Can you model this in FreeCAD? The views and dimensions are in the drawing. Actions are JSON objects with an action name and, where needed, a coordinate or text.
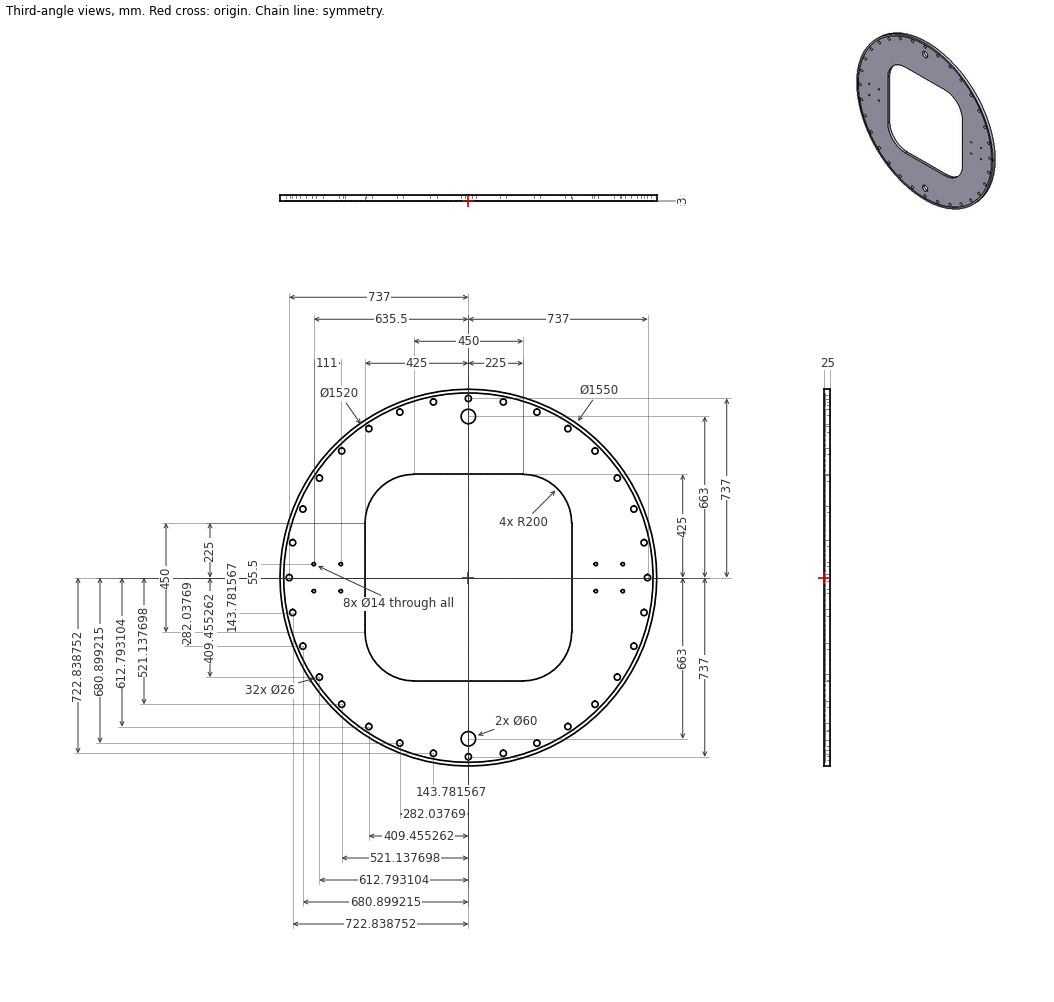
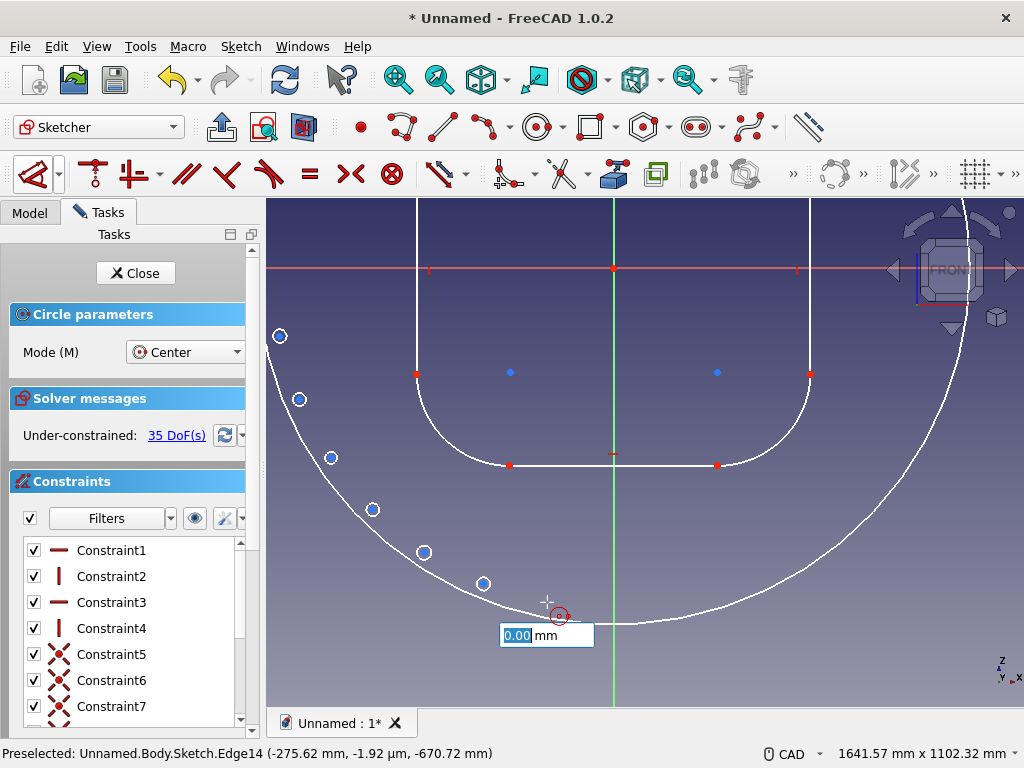
{"action": "scroll", "coordinate": [551, 598], "scroll_direction": "up", "scroll_amount": 5}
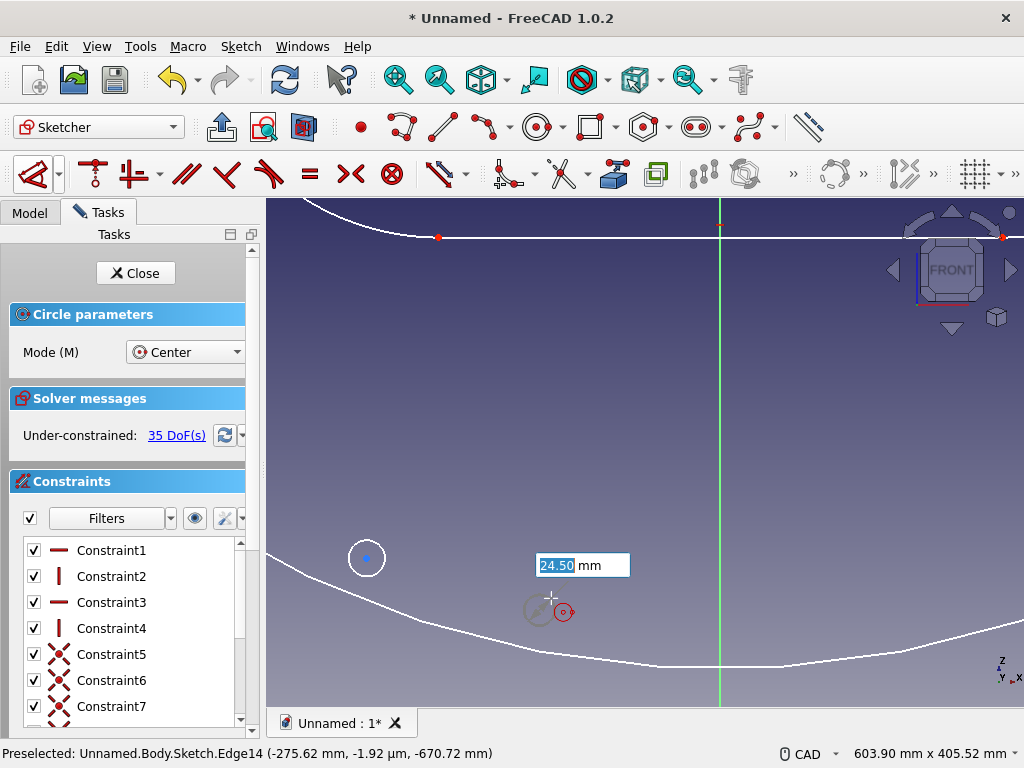
{"action": "left_click", "coordinate": [552, 596]}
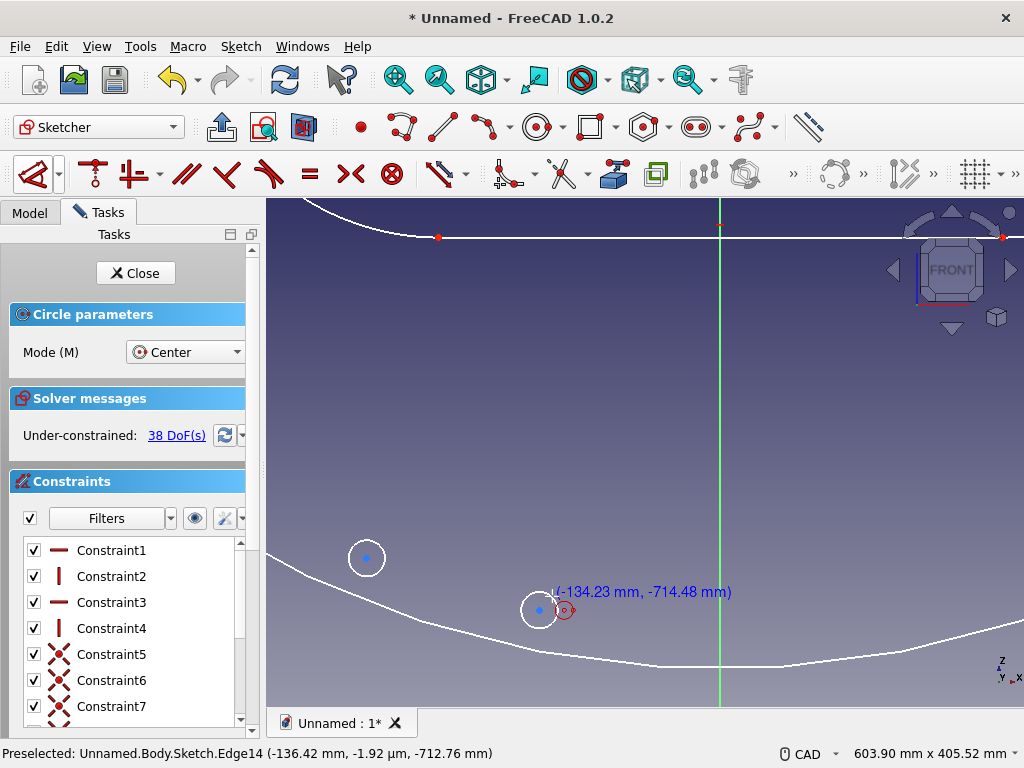
{"action": "scroll", "coordinate": [720, 625], "scroll_direction": "up", "scroll_amount": 2}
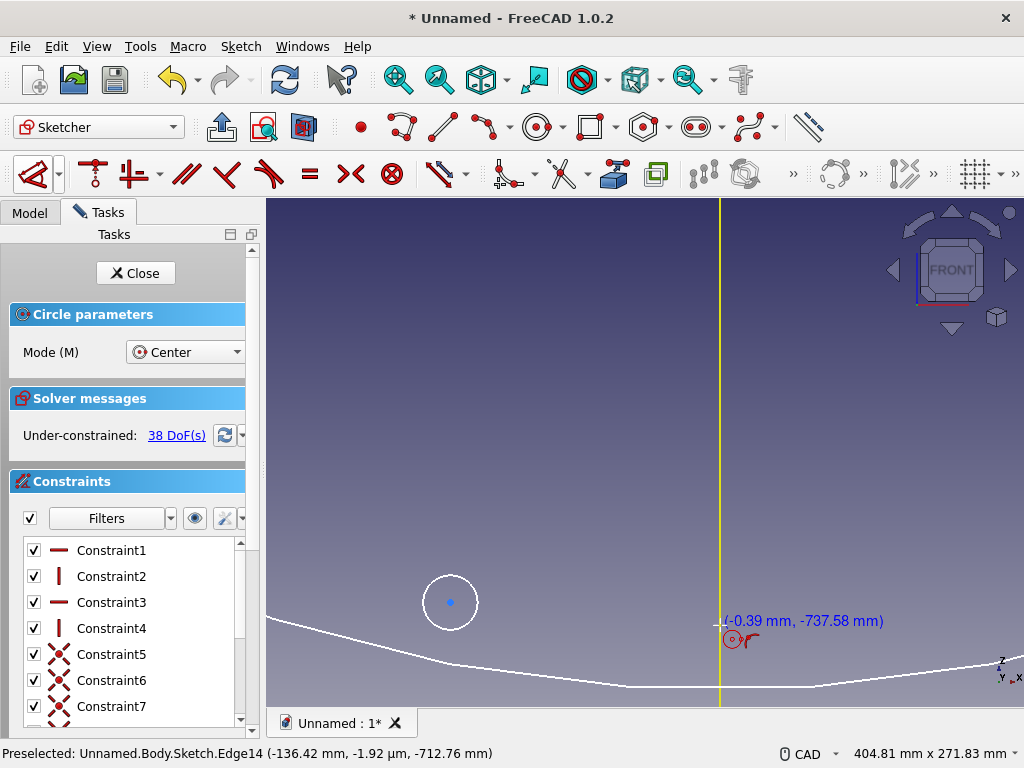
{"action": "scroll", "coordinate": [559, 603], "scroll_direction": "down", "scroll_amount": 11}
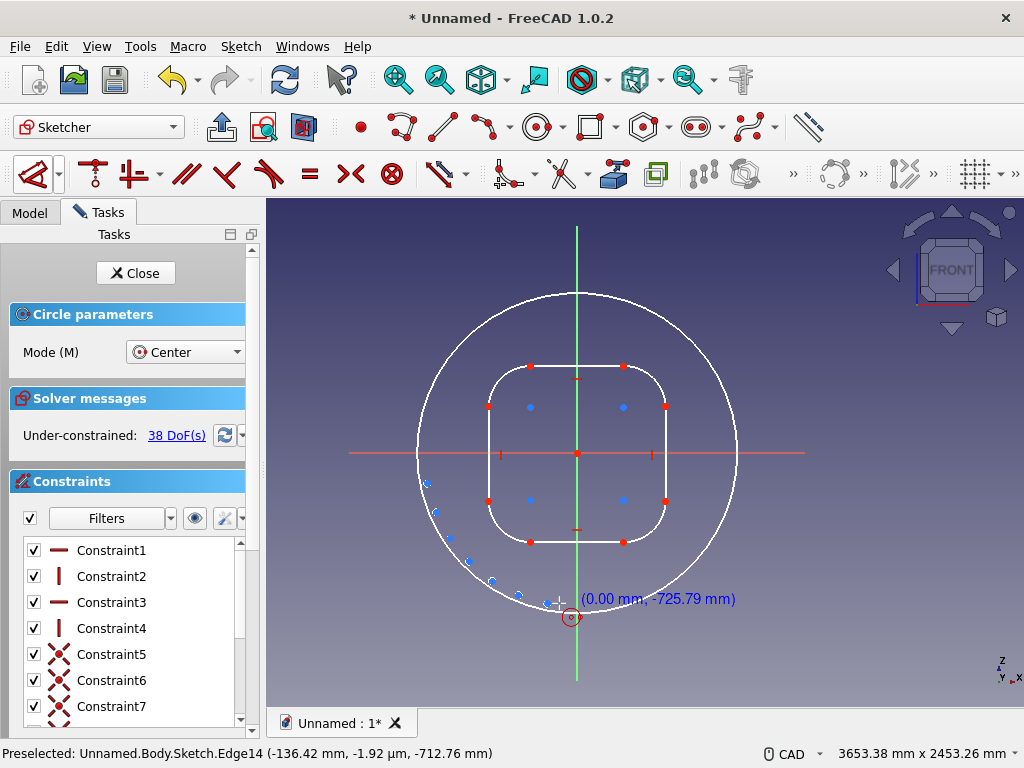
{"action": "scroll", "coordinate": [577, 606], "scroll_direction": "up", "scroll_amount": 4}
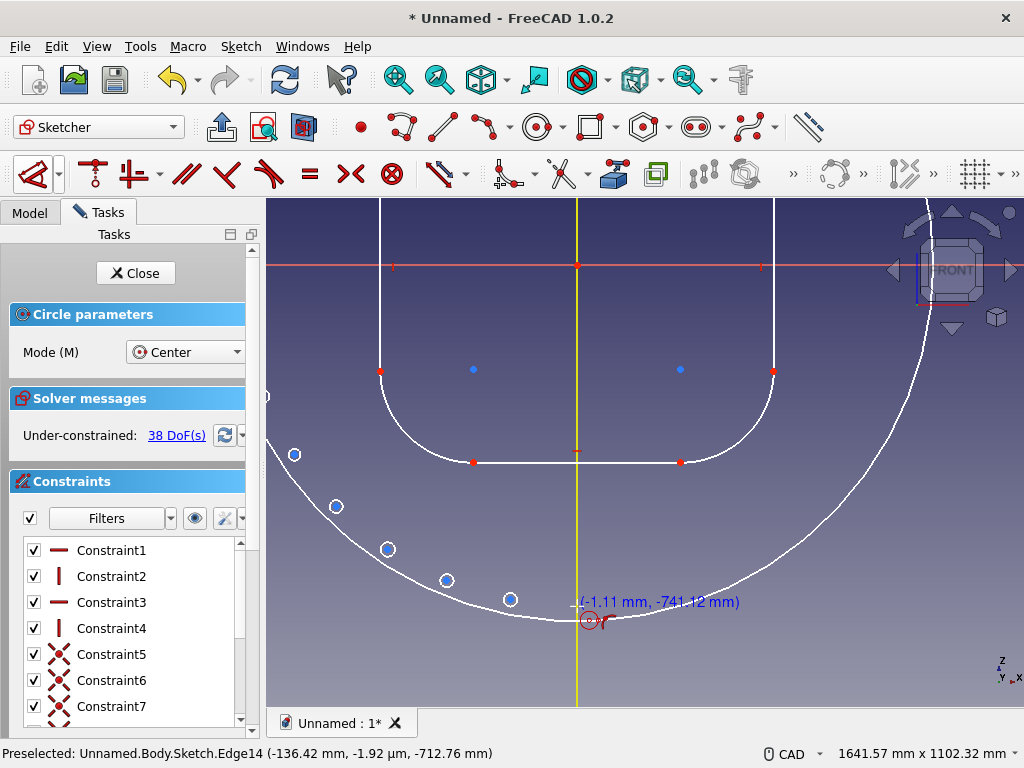
{"action": "left_click", "coordinate": [577, 605]}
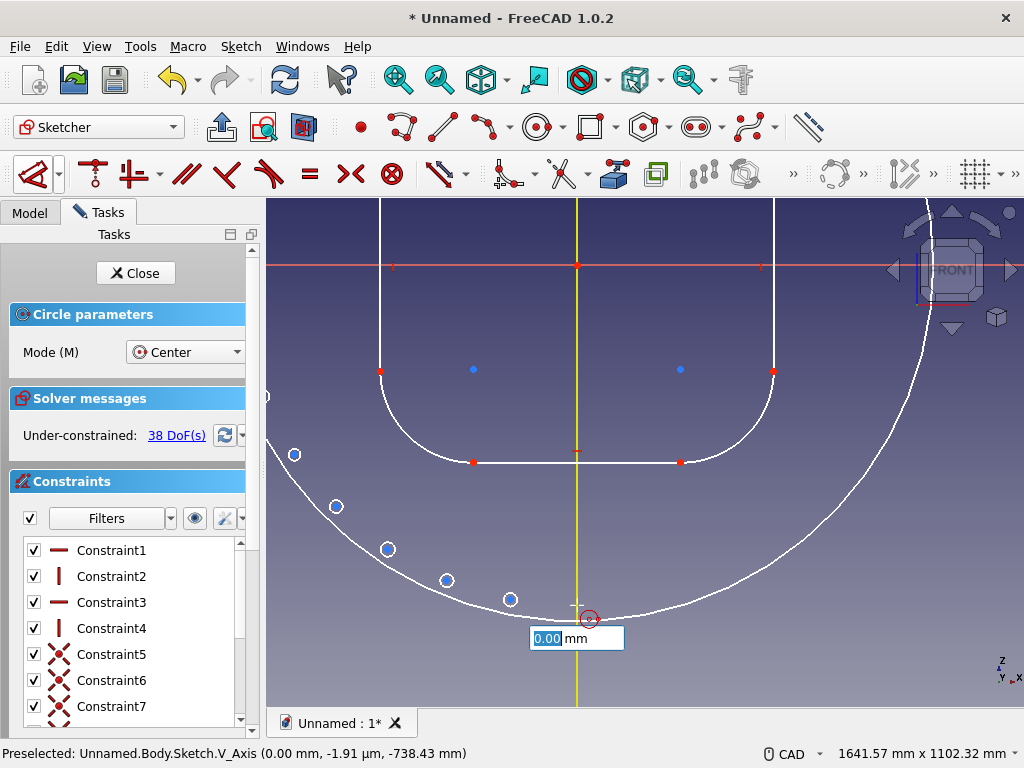
{"action": "scroll", "coordinate": [583, 603], "scroll_direction": "up", "scroll_amount": 6}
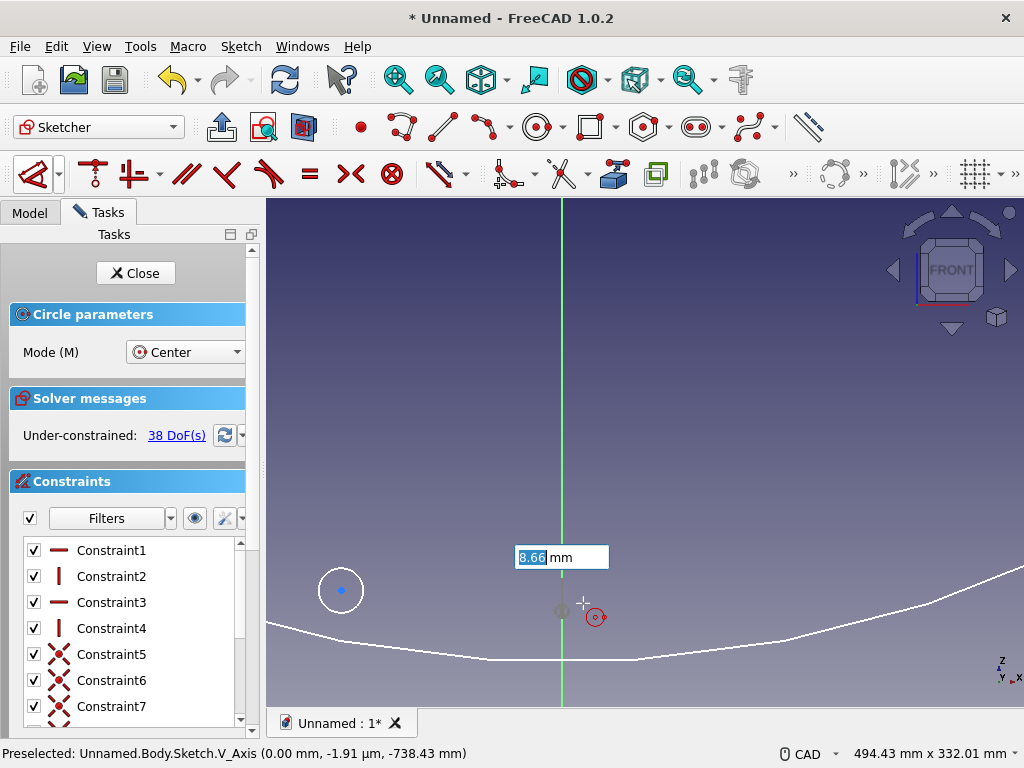
{"action": "left_click", "coordinate": [581, 602]}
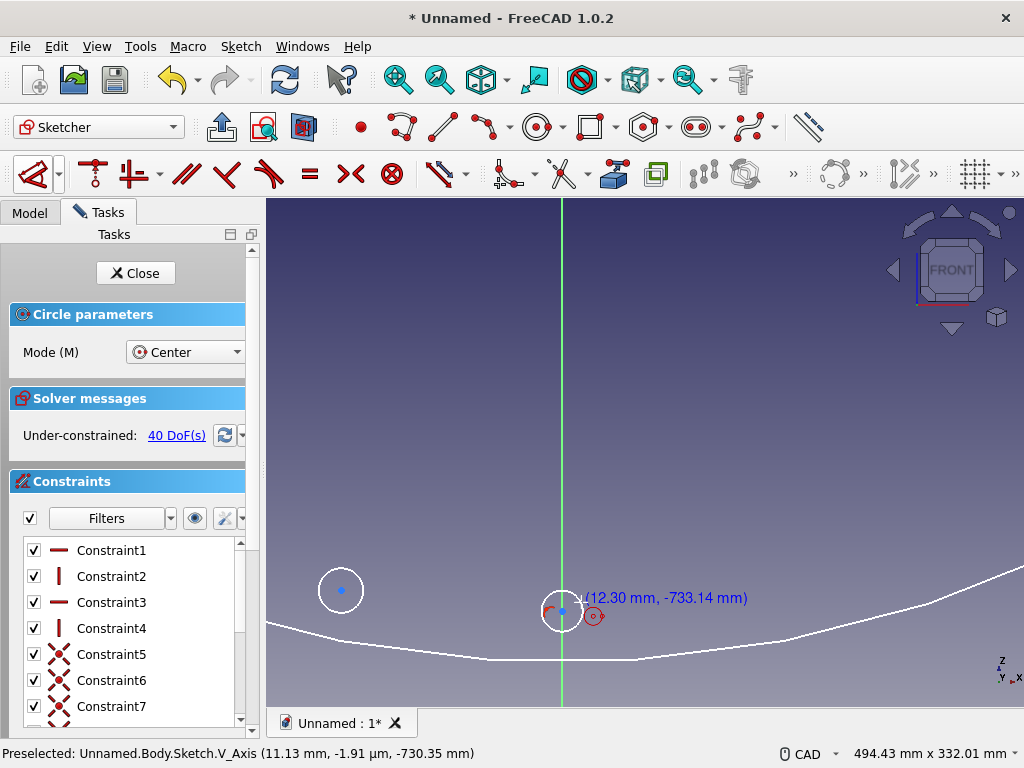
{"action": "scroll", "coordinate": [579, 605], "scroll_direction": "down", "scroll_amount": 10}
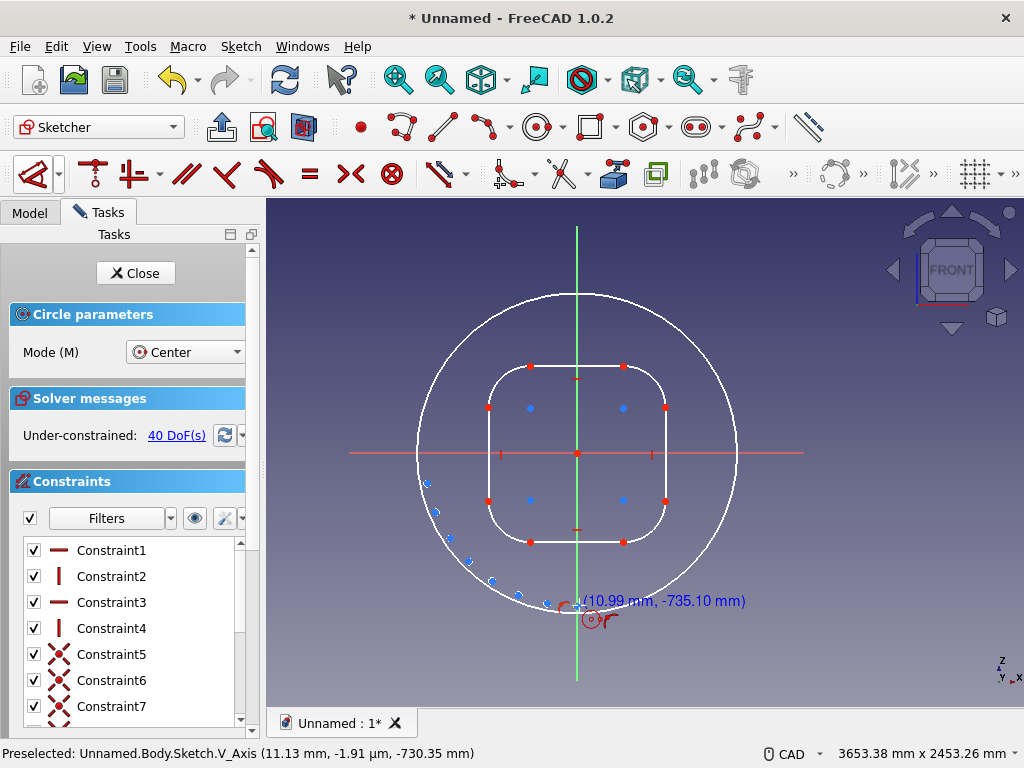
{"action": "scroll", "coordinate": [577, 591], "scroll_direction": "up", "scroll_amount": 2}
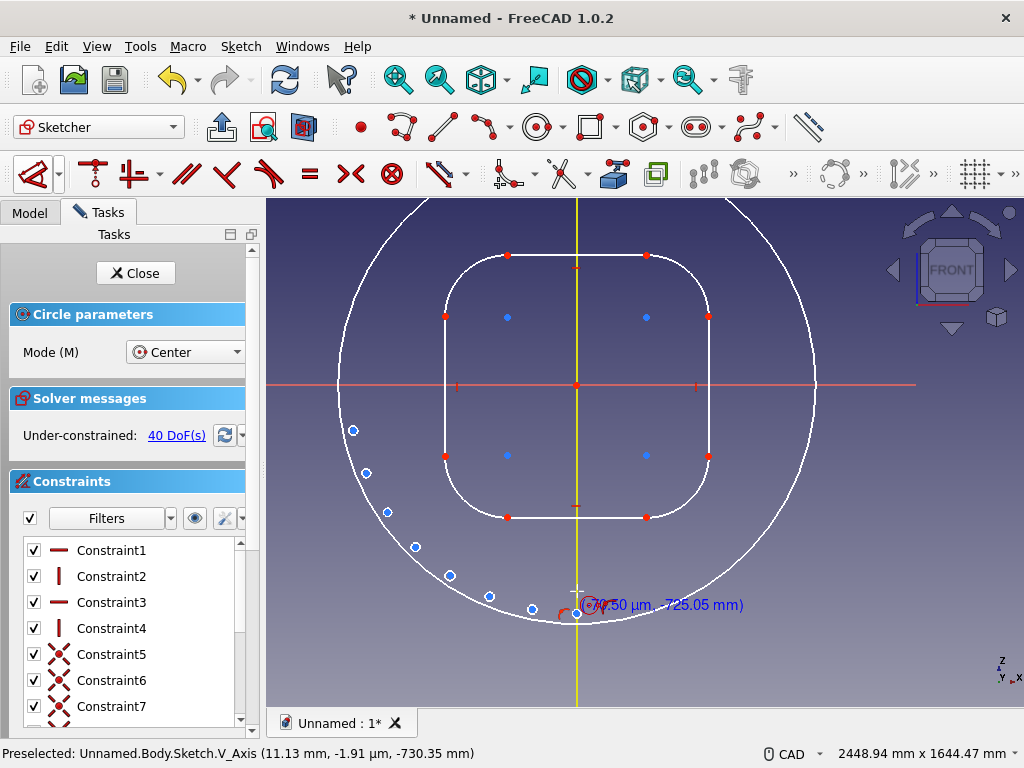
{"action": "left_click", "coordinate": [577, 590]}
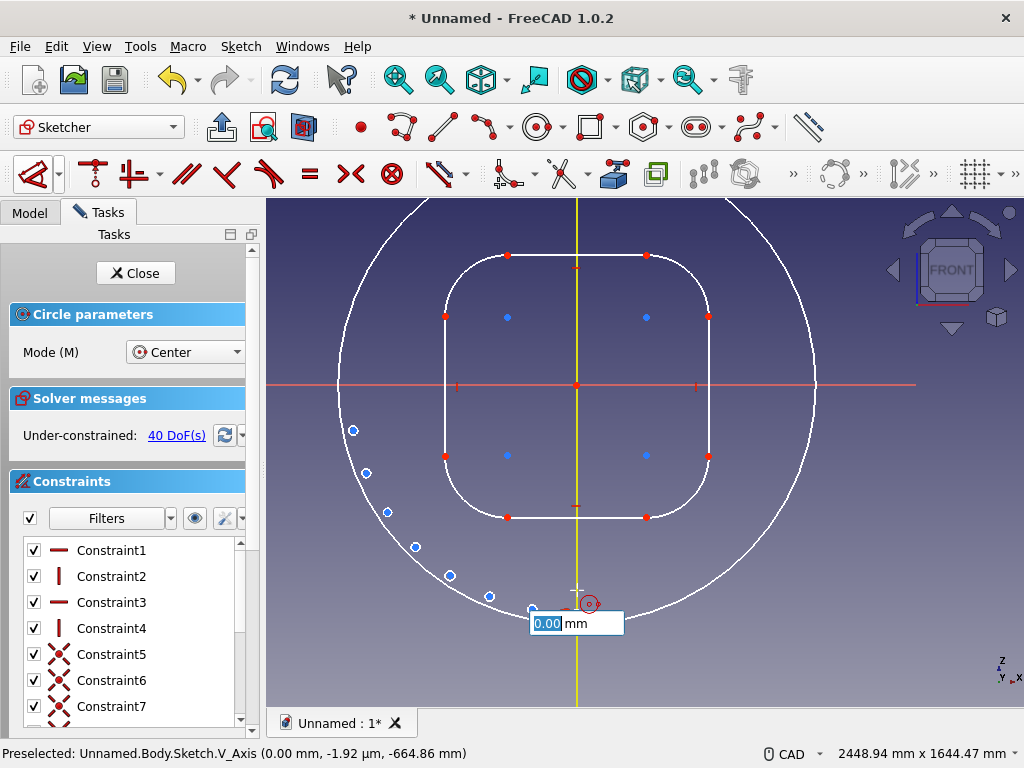
{"action": "scroll", "coordinate": [586, 587], "scroll_direction": "up", "scroll_amount": 3}